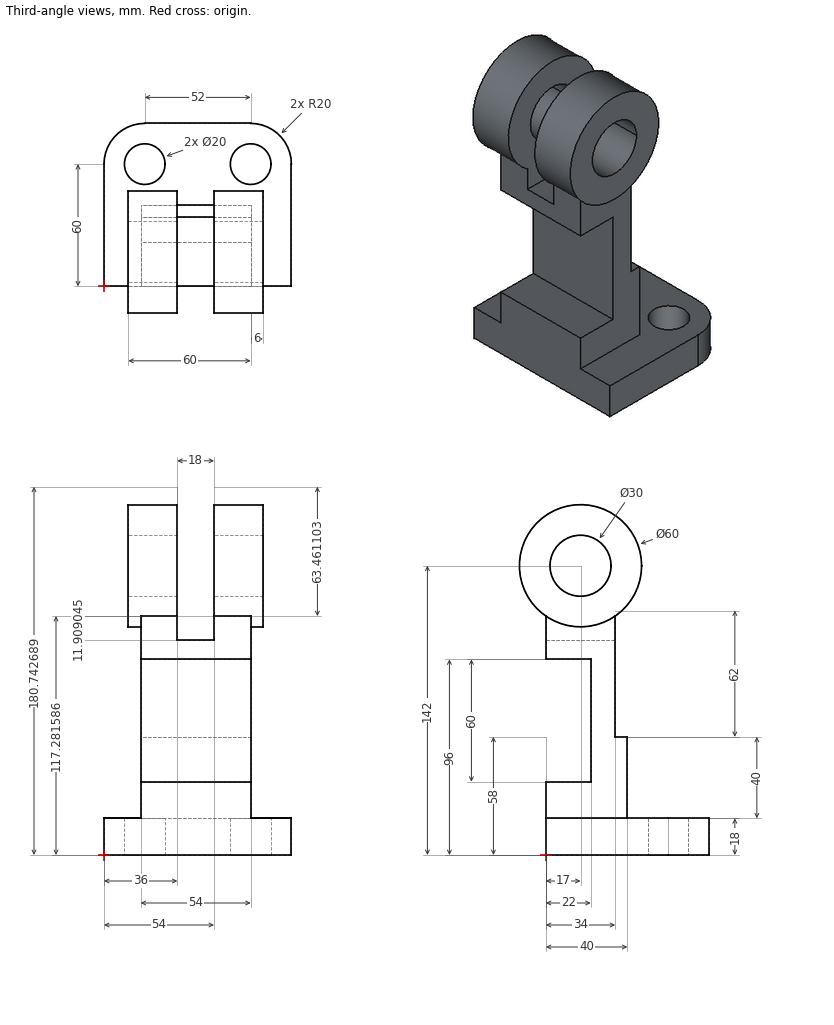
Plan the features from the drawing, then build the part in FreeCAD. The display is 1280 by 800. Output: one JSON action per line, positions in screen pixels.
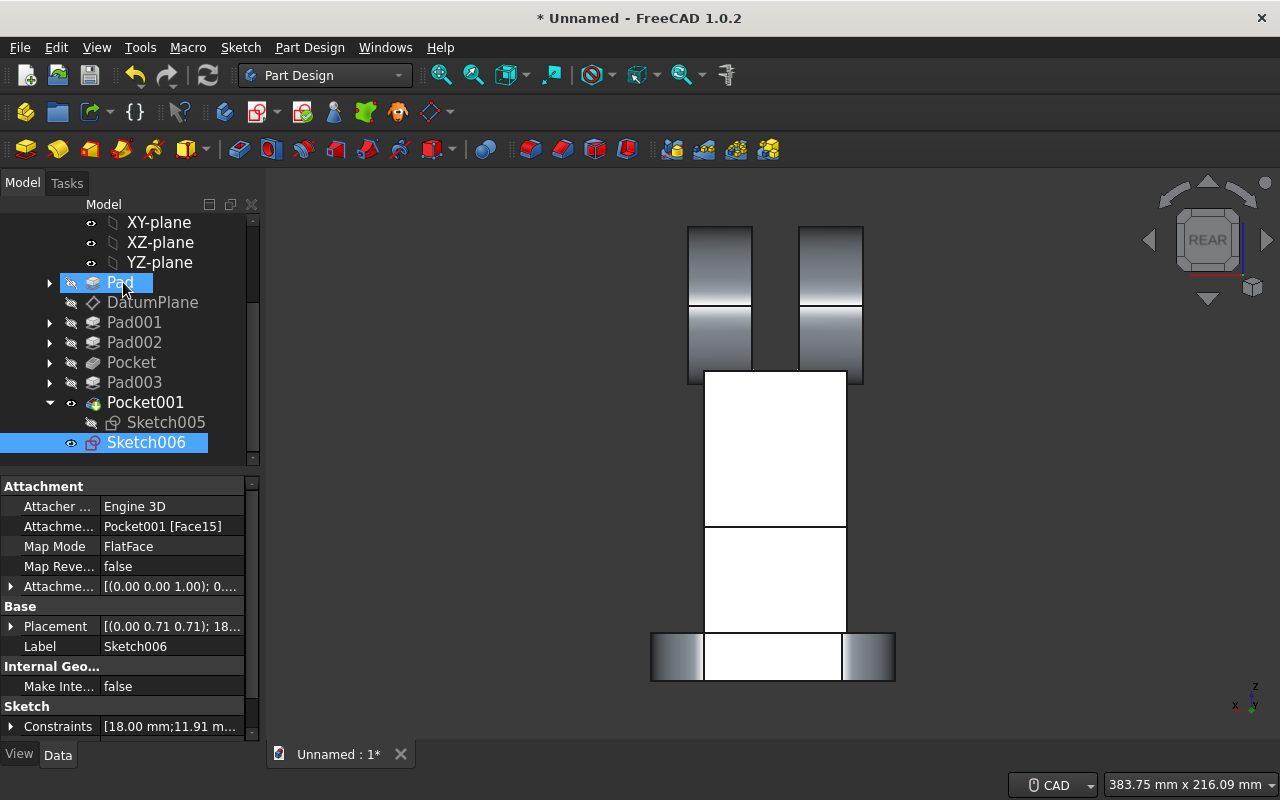
{"action": "left_click", "coordinate": [240, 150]}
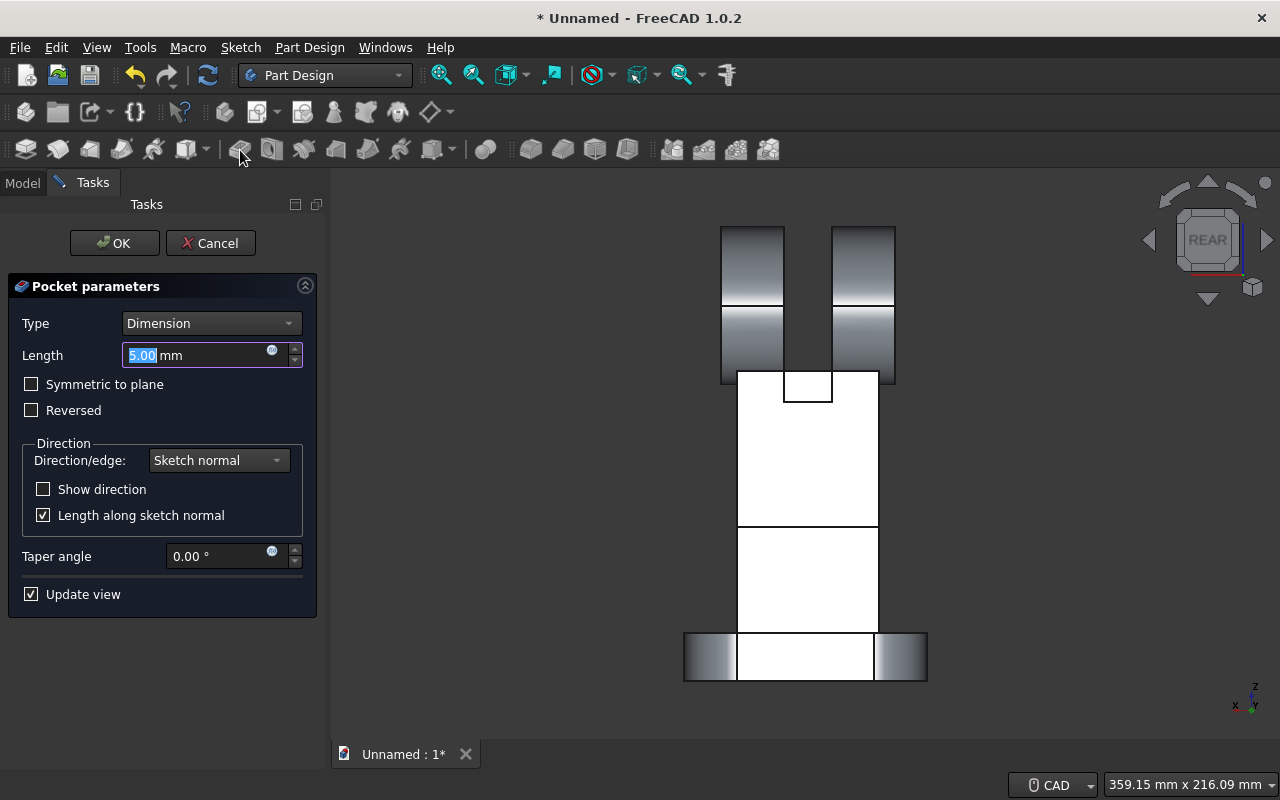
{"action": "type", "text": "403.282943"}
{"action": "key", "text": "Tab"}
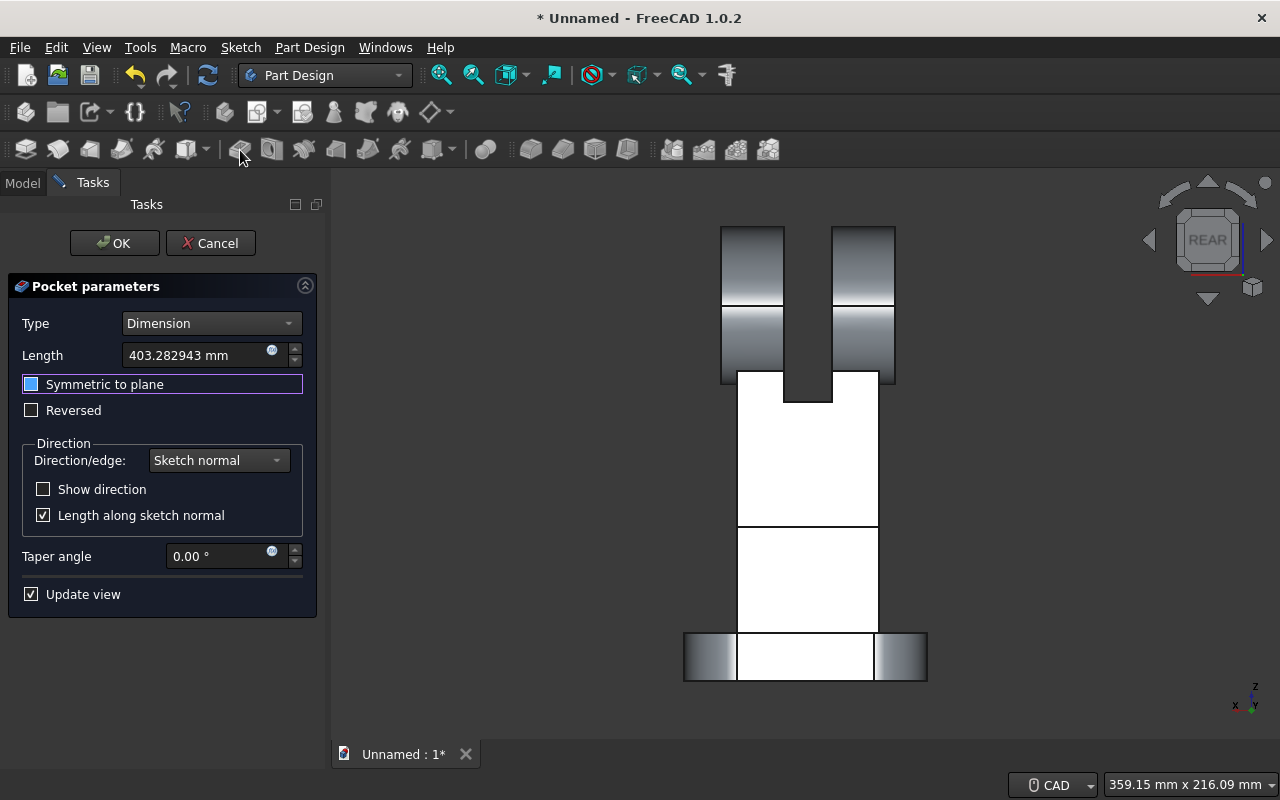
{"action": "left_click", "coordinate": [30, 384]}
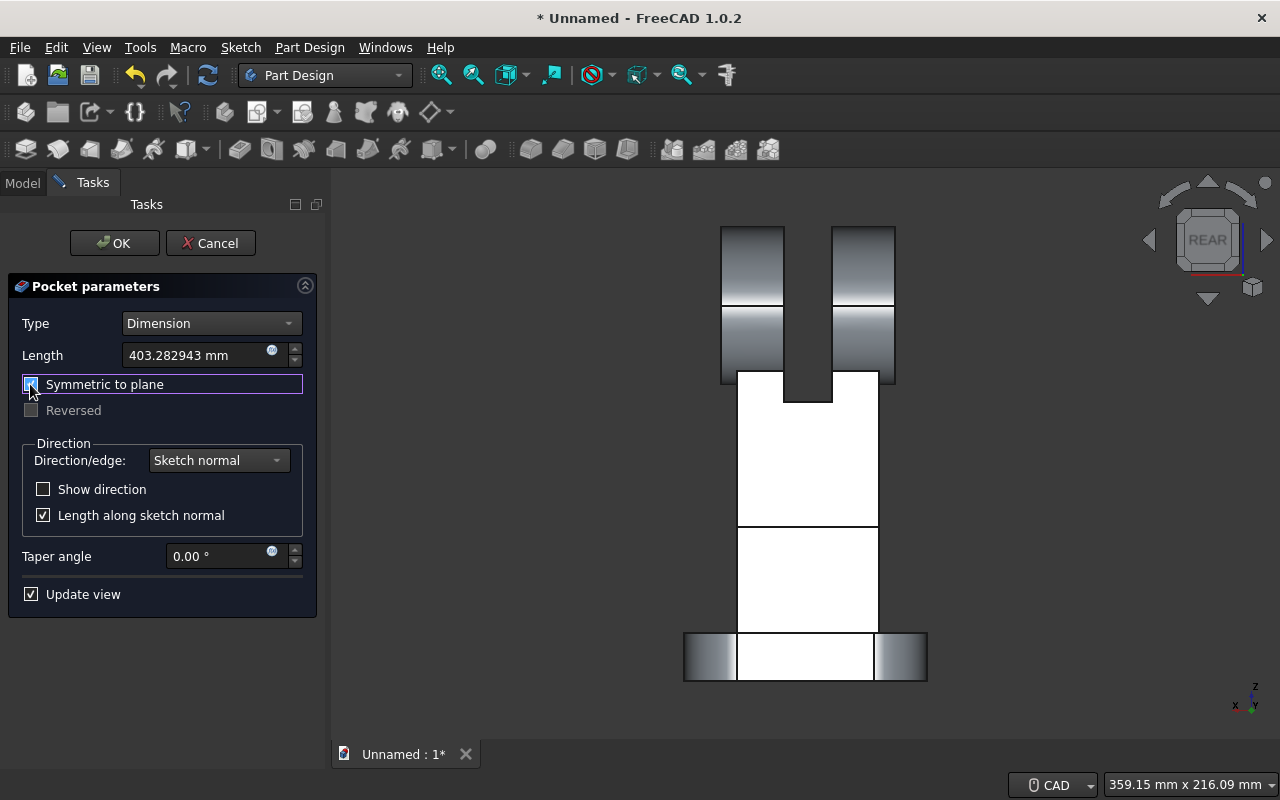
{"action": "left_click", "coordinate": [115, 243]}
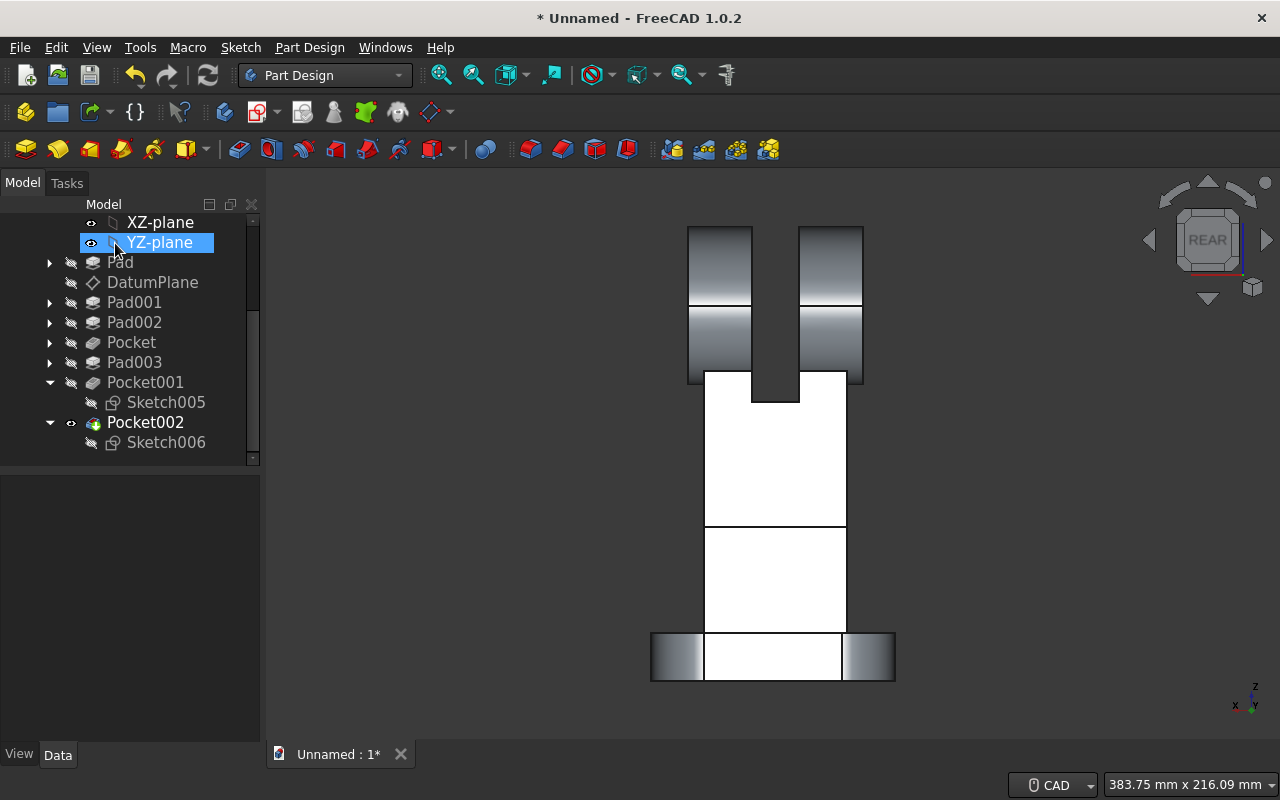
{"action": "key", "text": "0"}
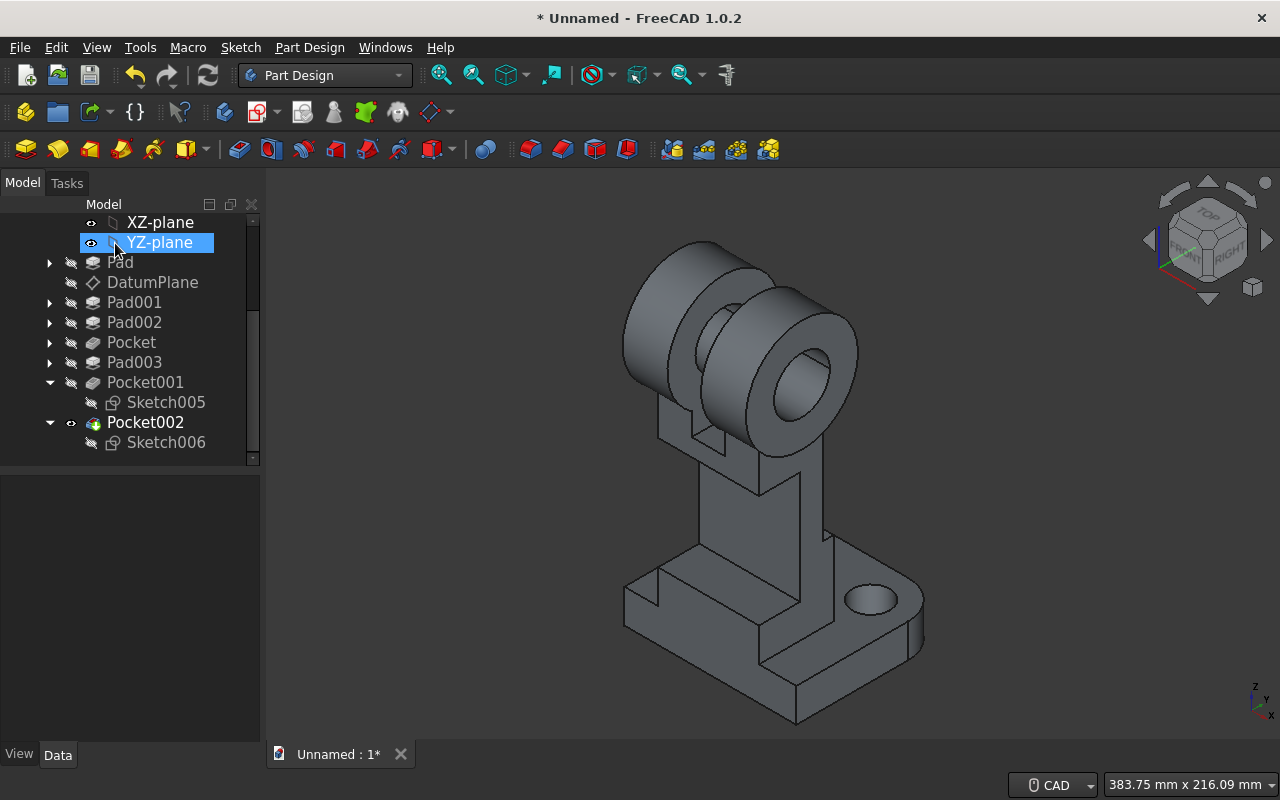
{"action": "left_click", "coordinate": [442, 76]}